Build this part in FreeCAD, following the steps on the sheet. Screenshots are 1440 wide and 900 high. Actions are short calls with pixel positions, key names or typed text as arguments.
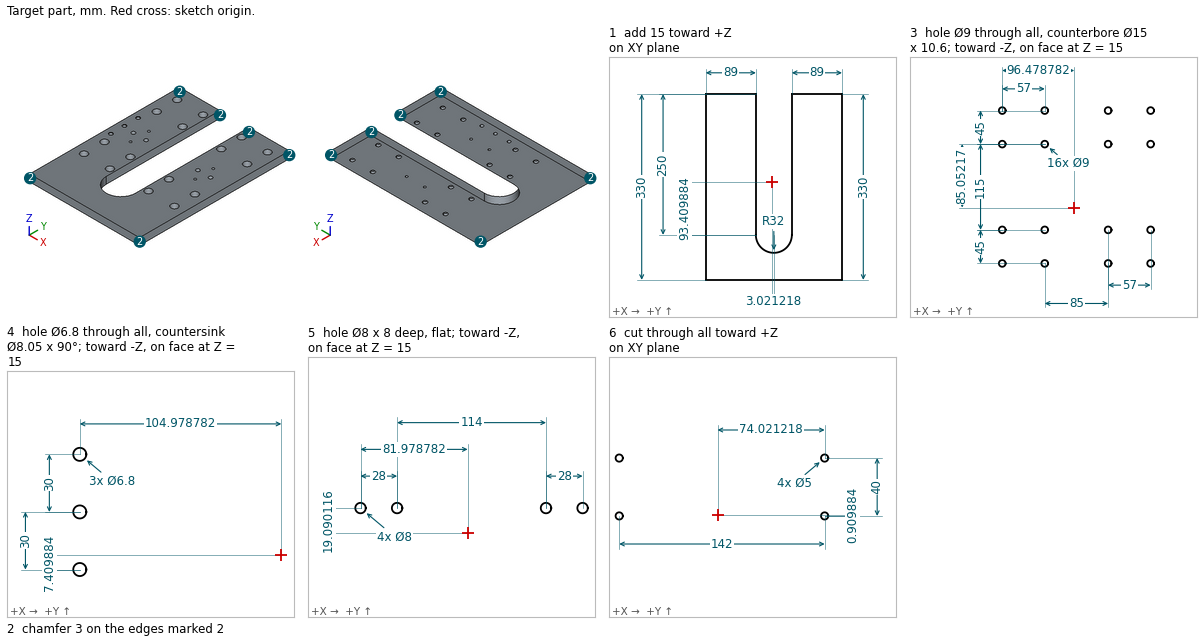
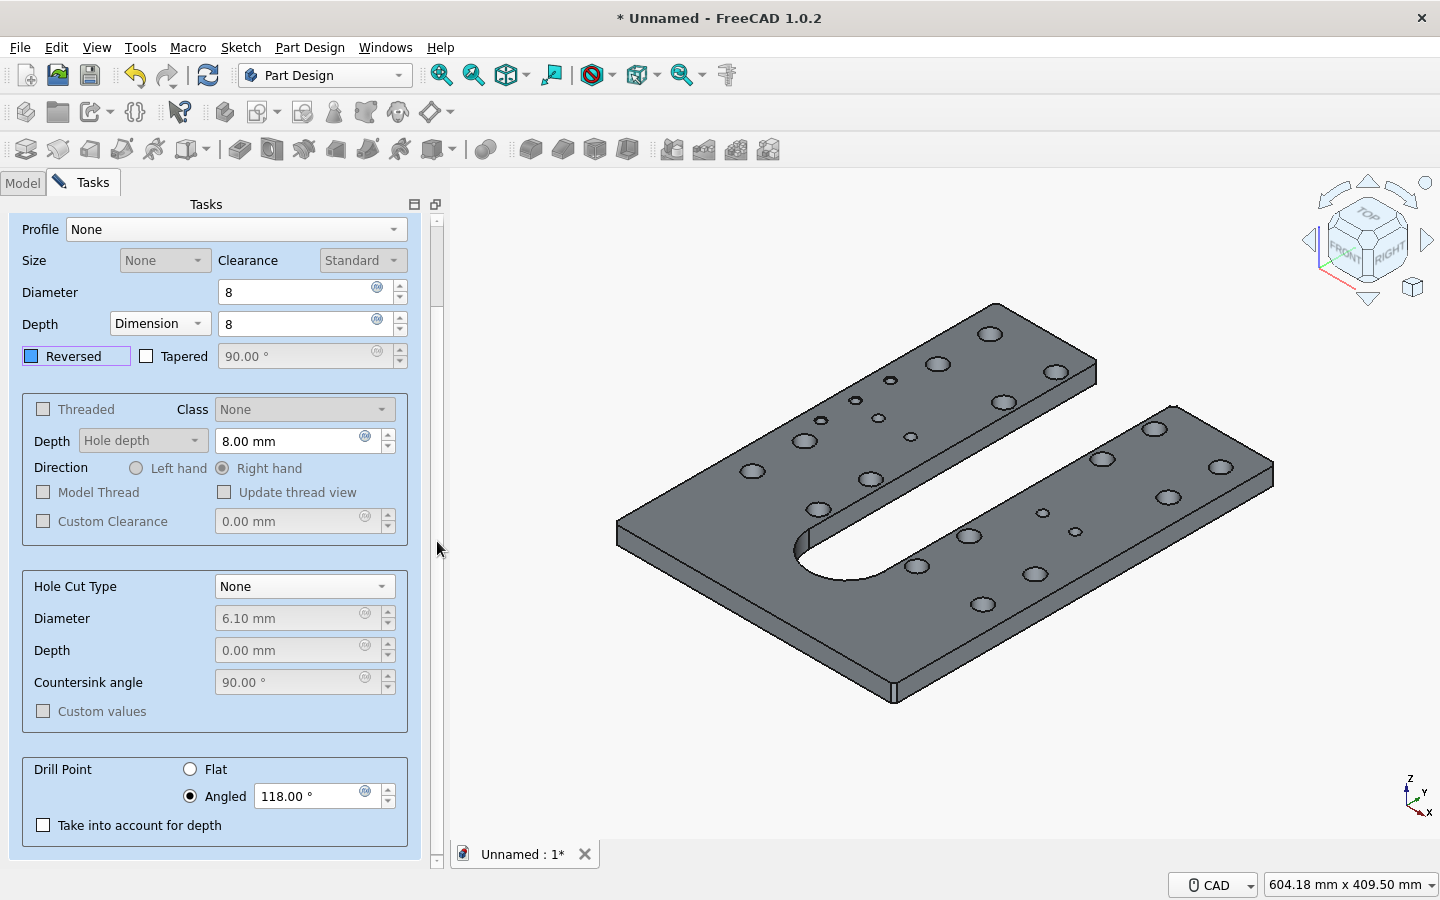
click(191, 769)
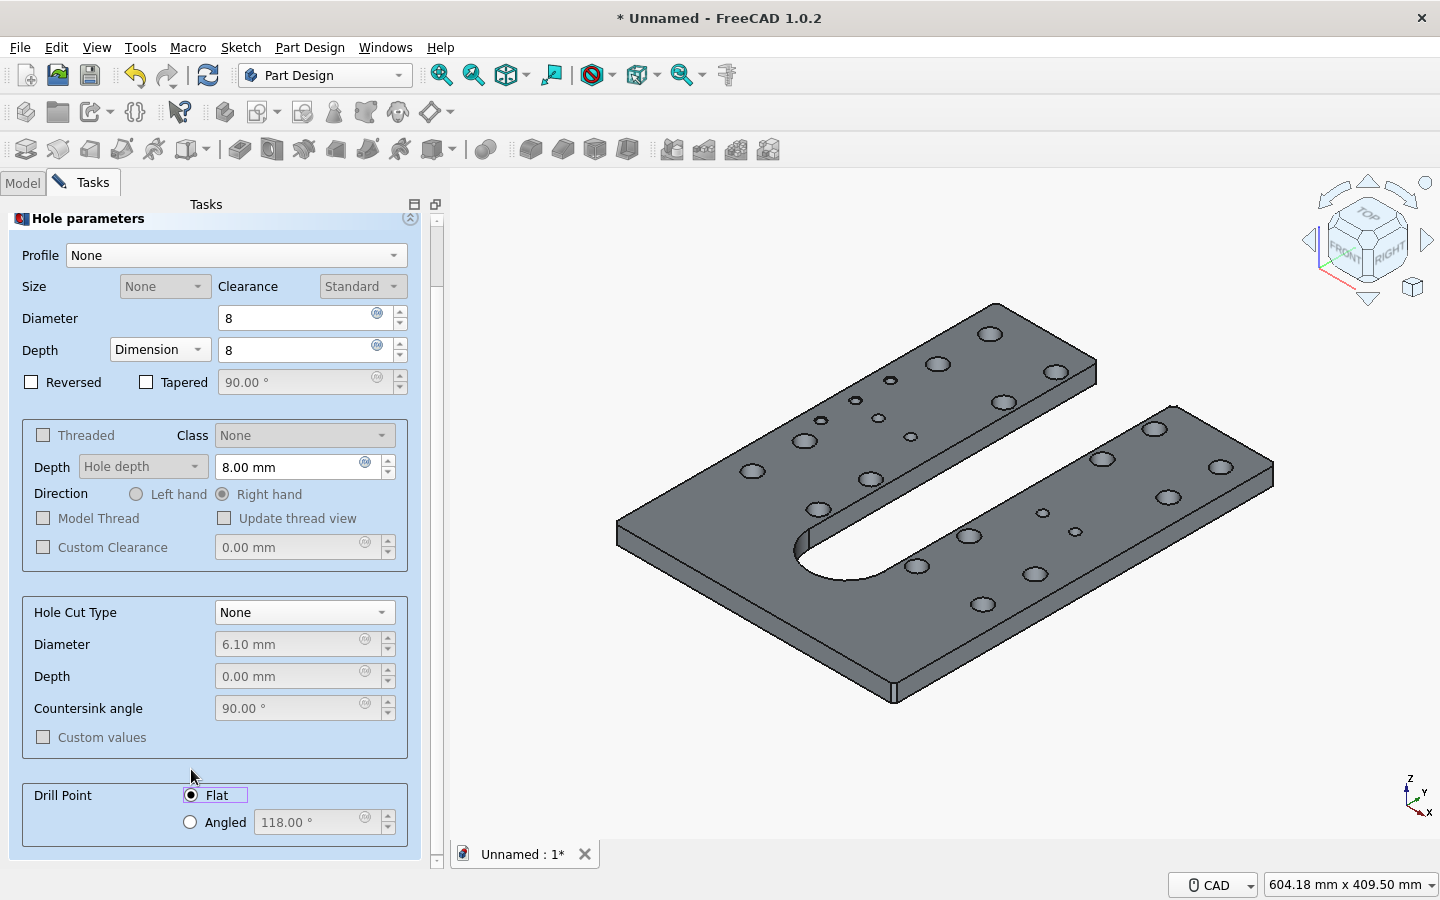
scroll(437, 541, up, 2)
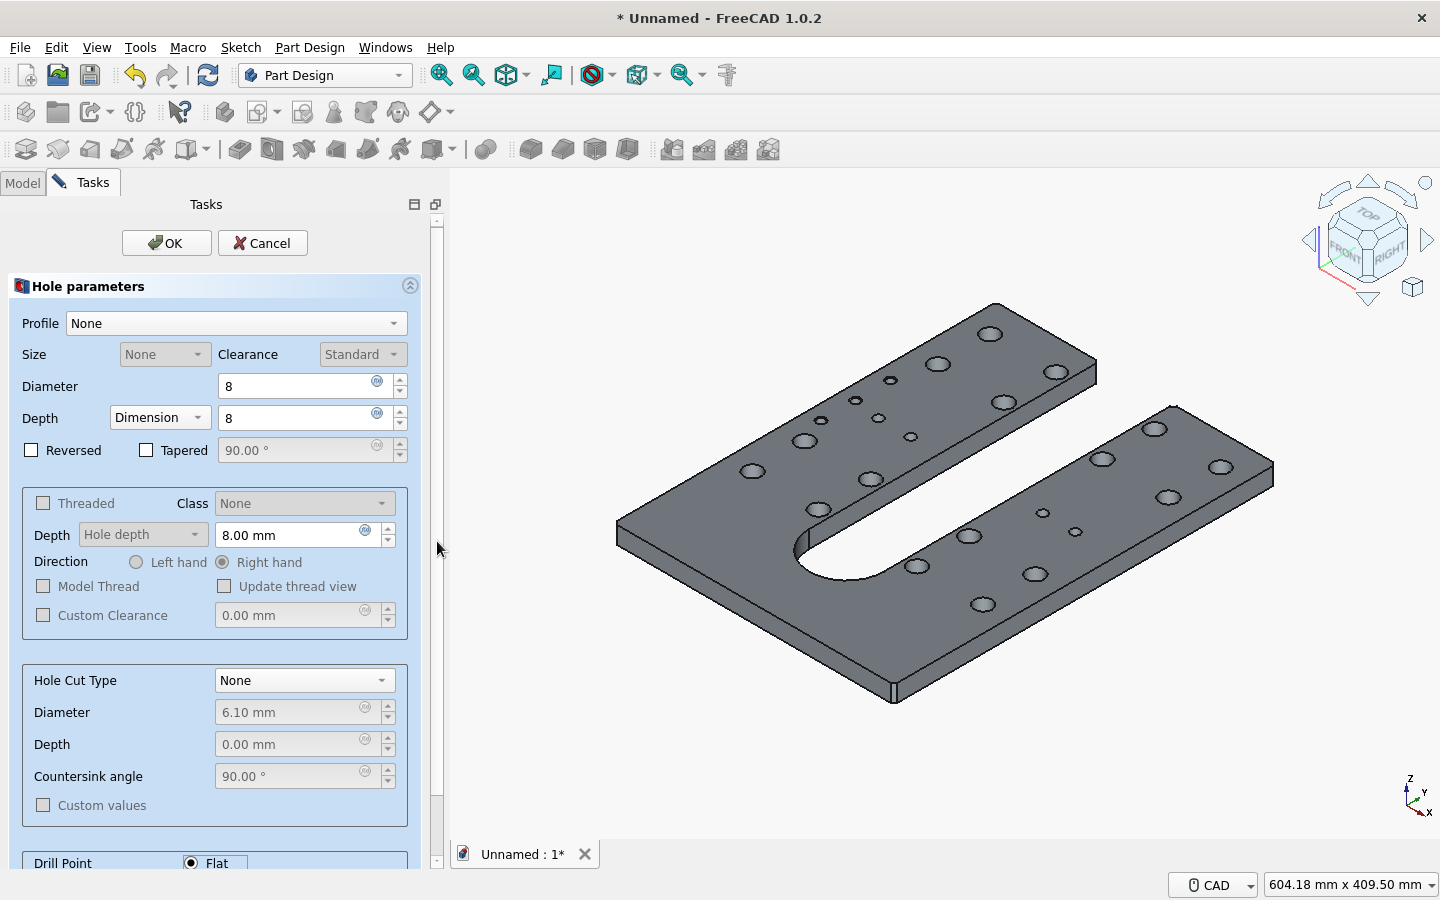
click(167, 243)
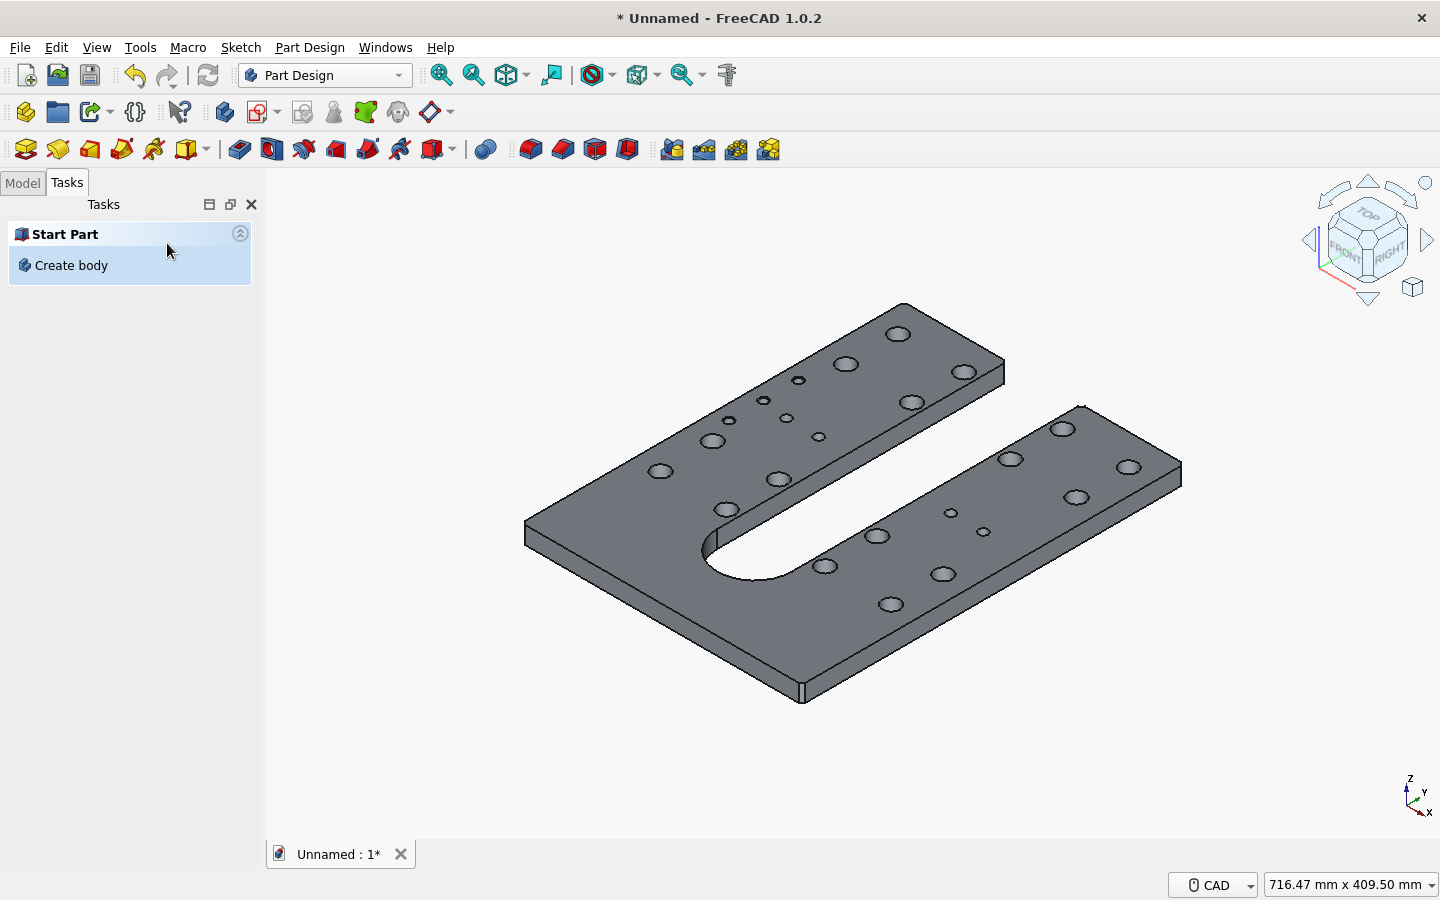
click(258, 112)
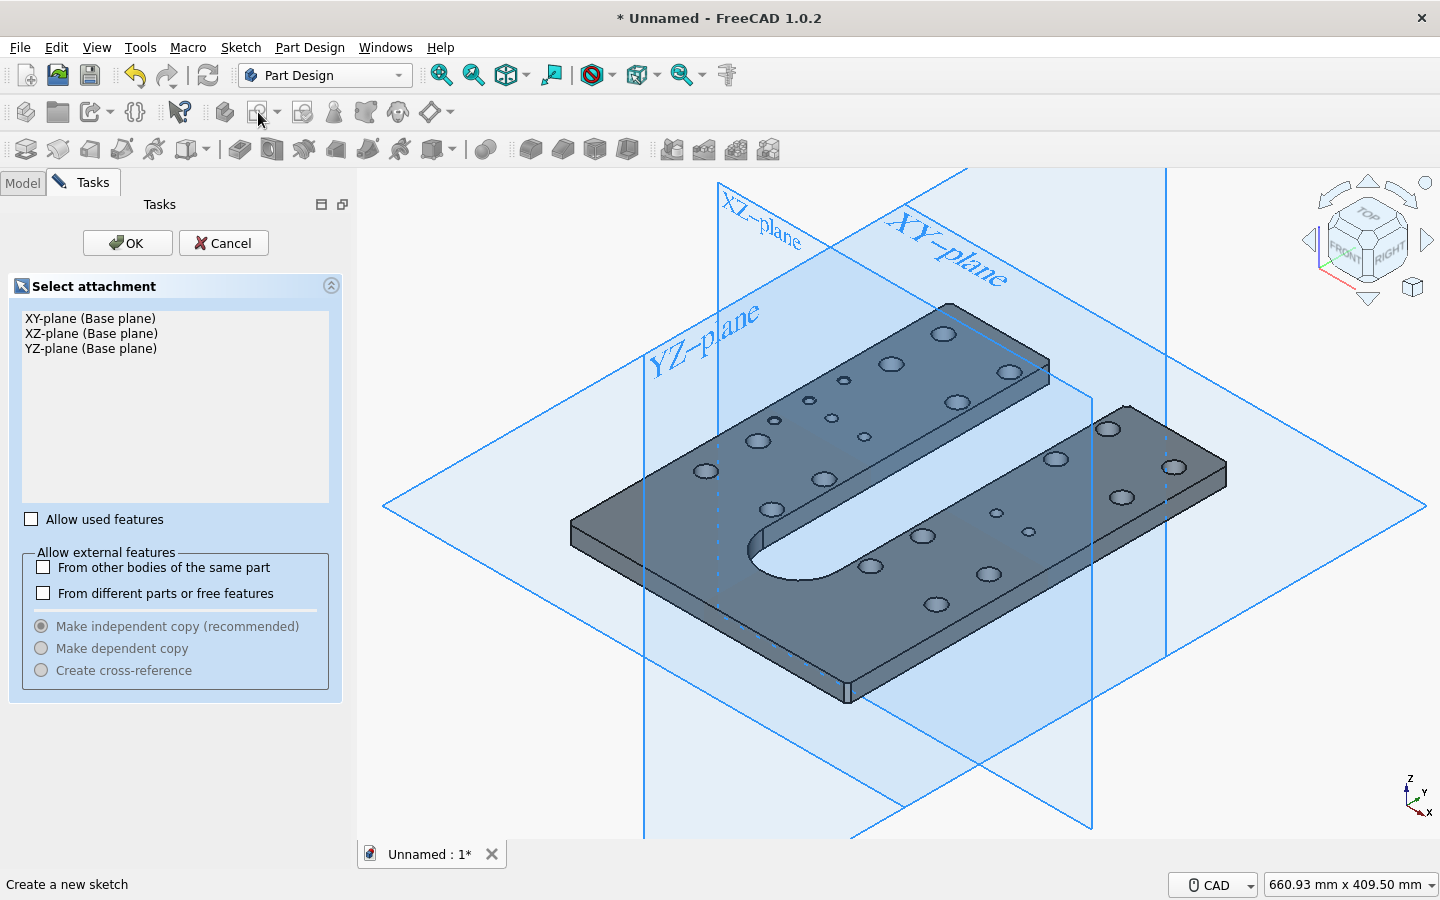
click(82, 318)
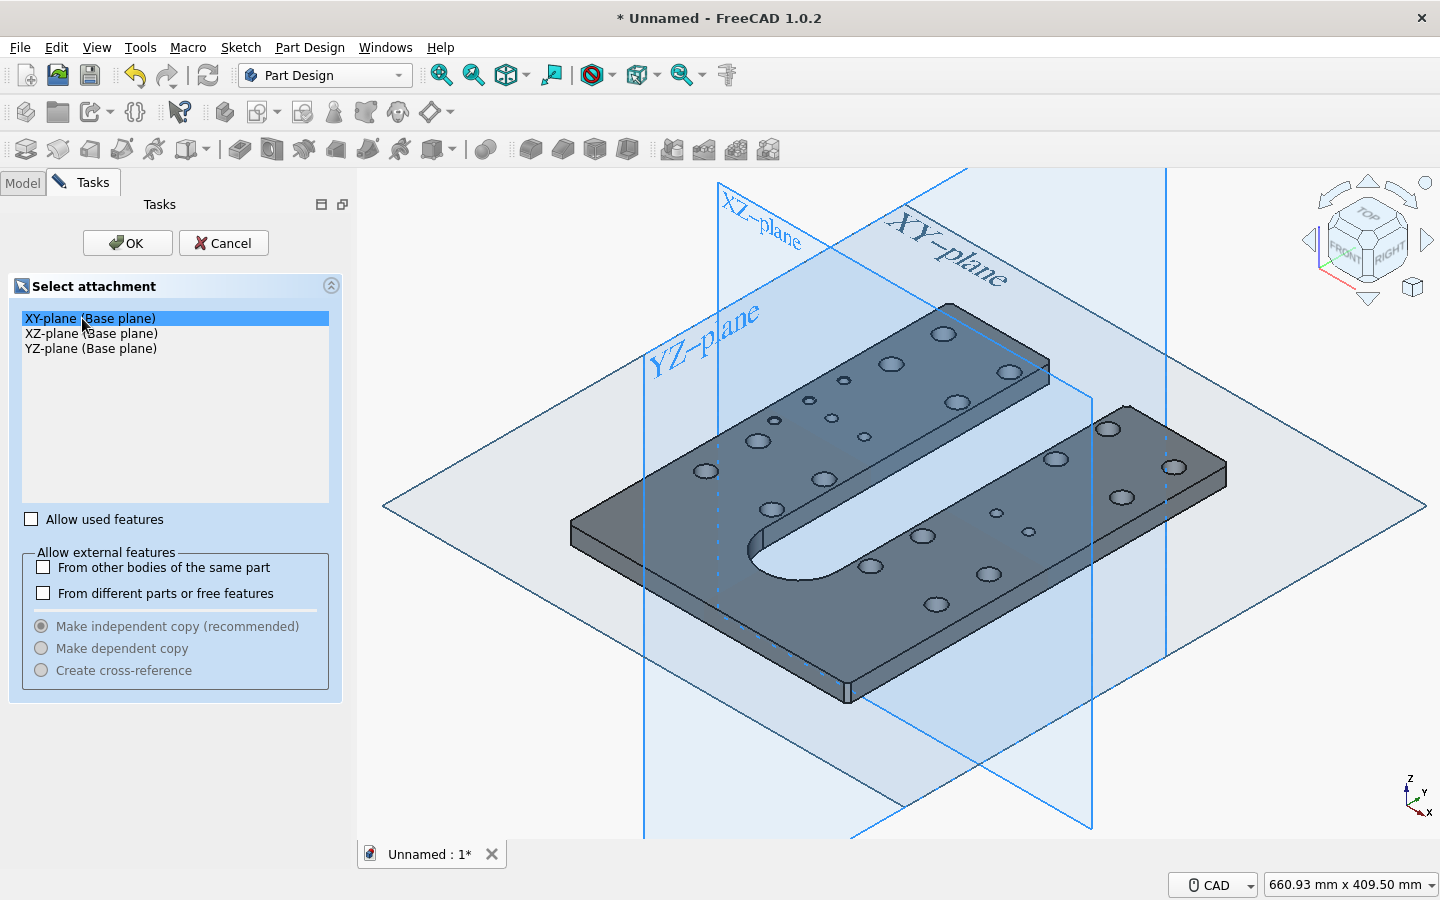
click(128, 243)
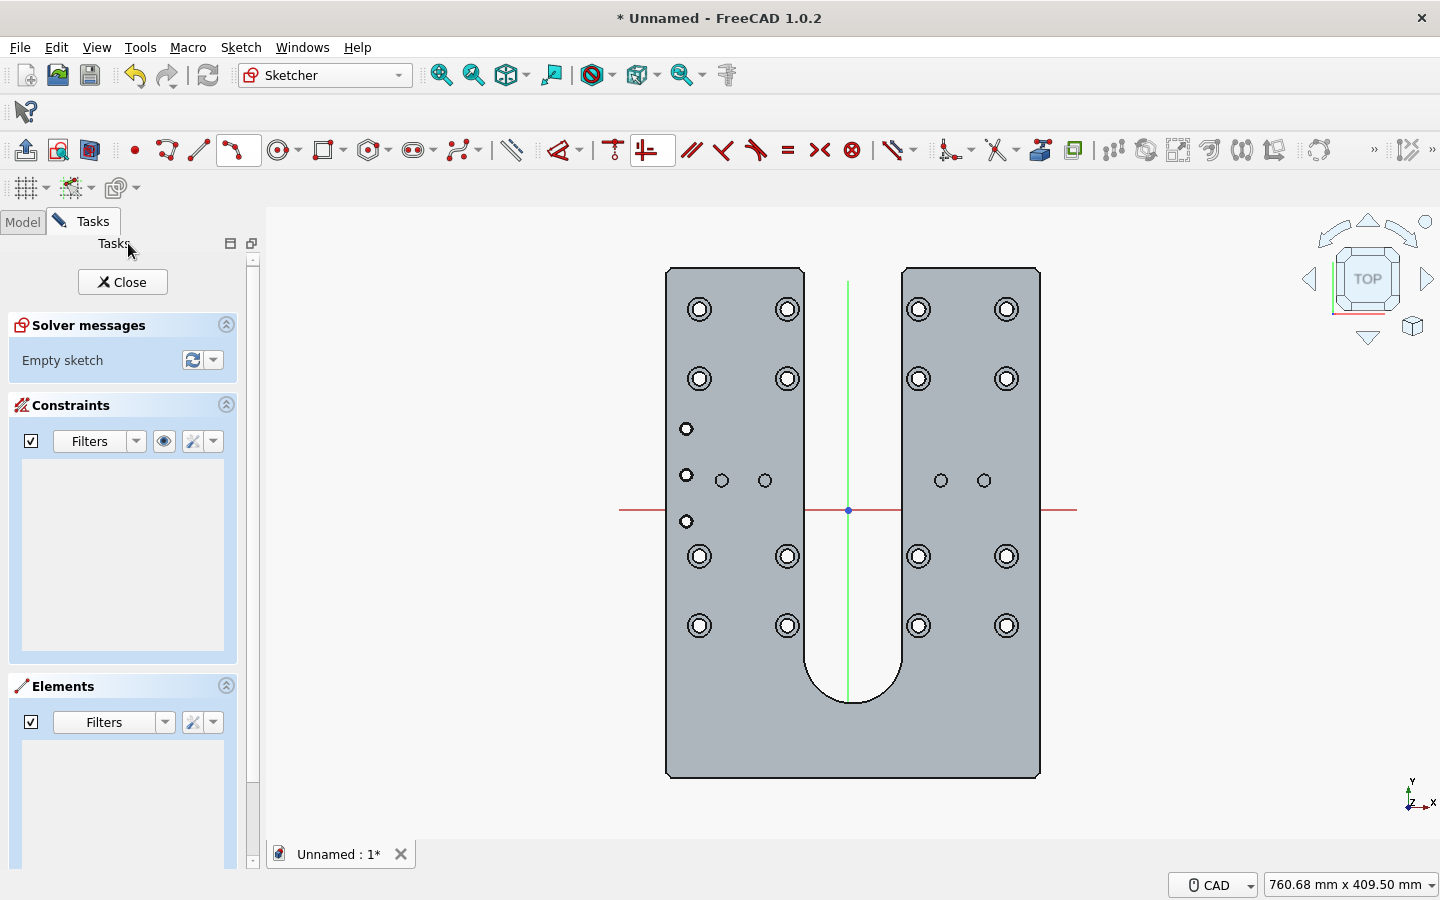
click(90, 150)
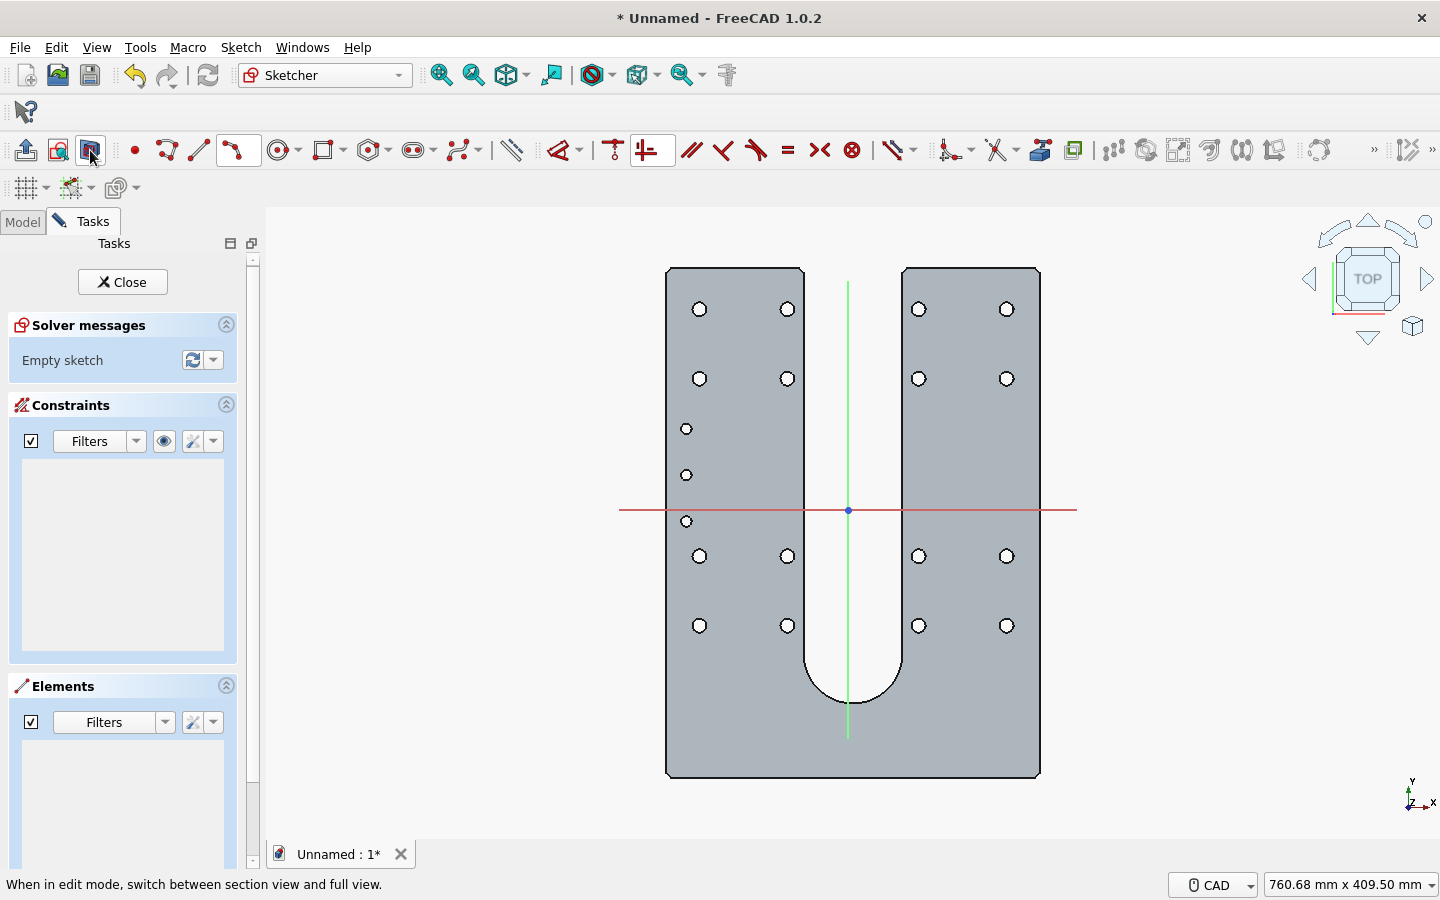
scroll(883, 462, up, 6)